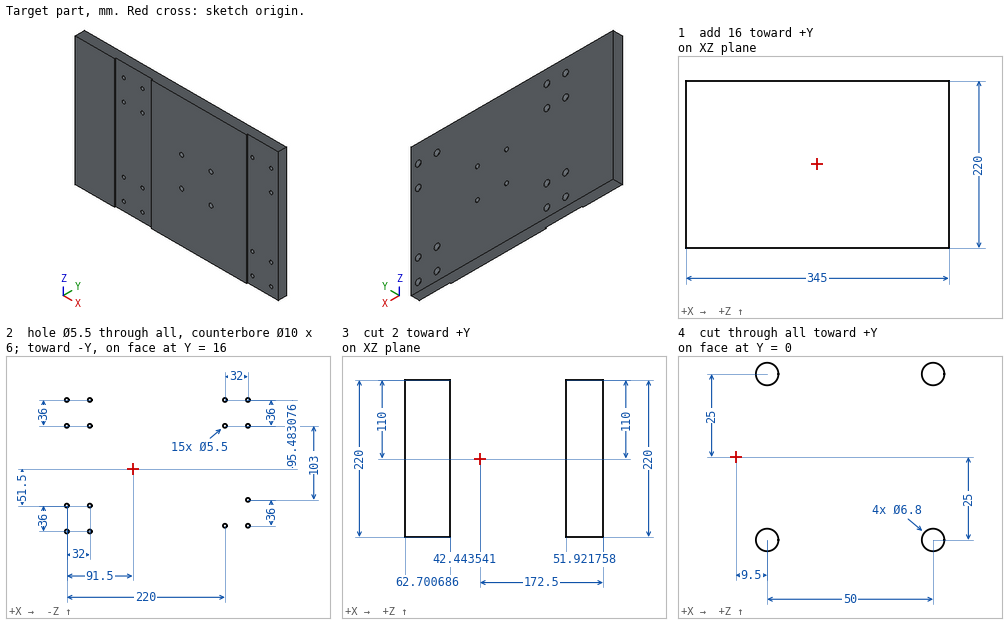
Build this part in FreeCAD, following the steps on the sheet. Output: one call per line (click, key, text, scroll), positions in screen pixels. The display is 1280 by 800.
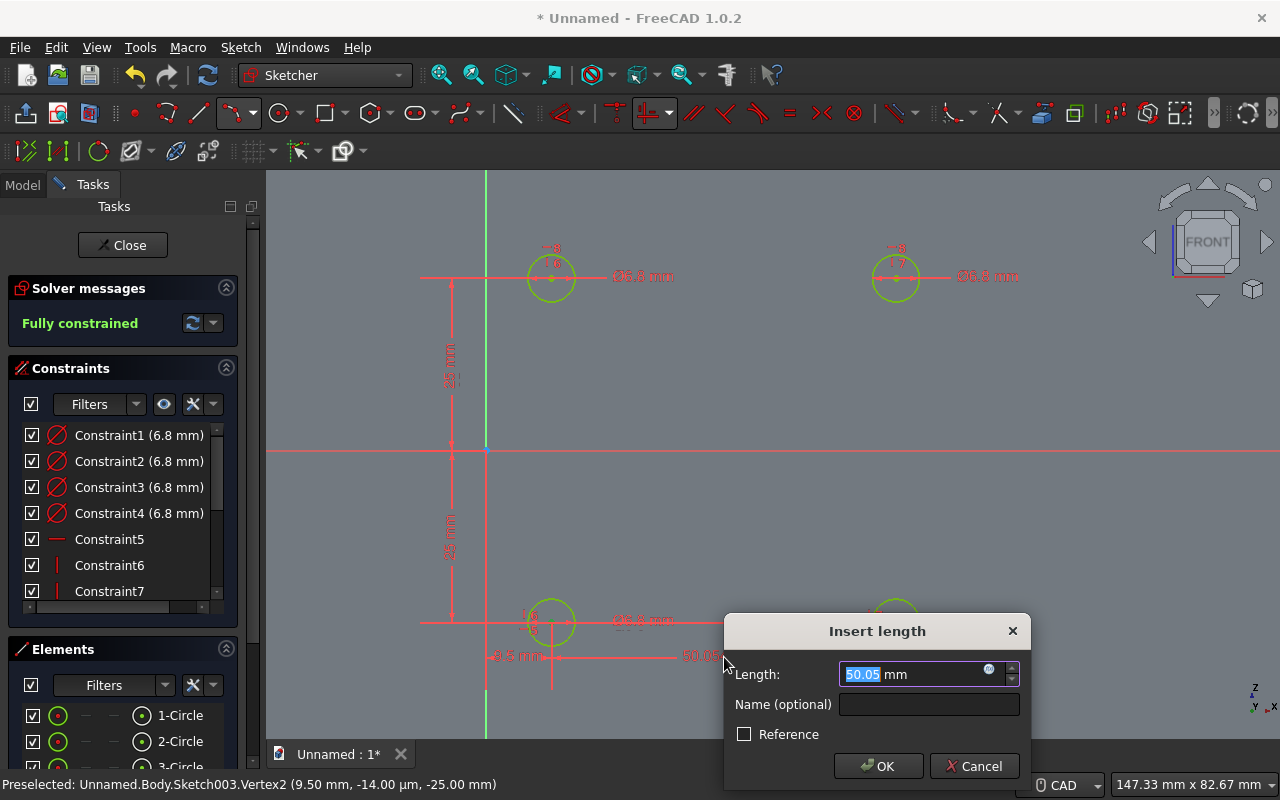
text(50)
key(Return)
key(Escape)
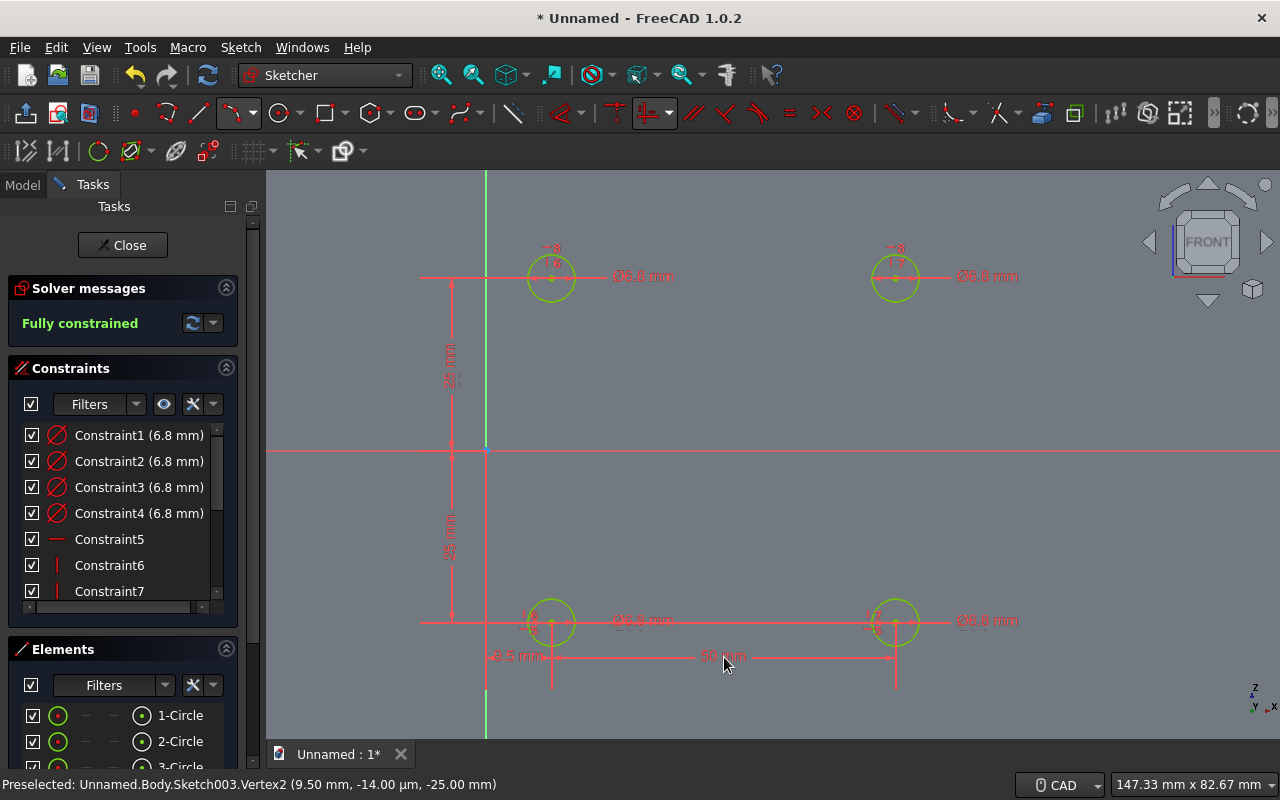
click(123, 245)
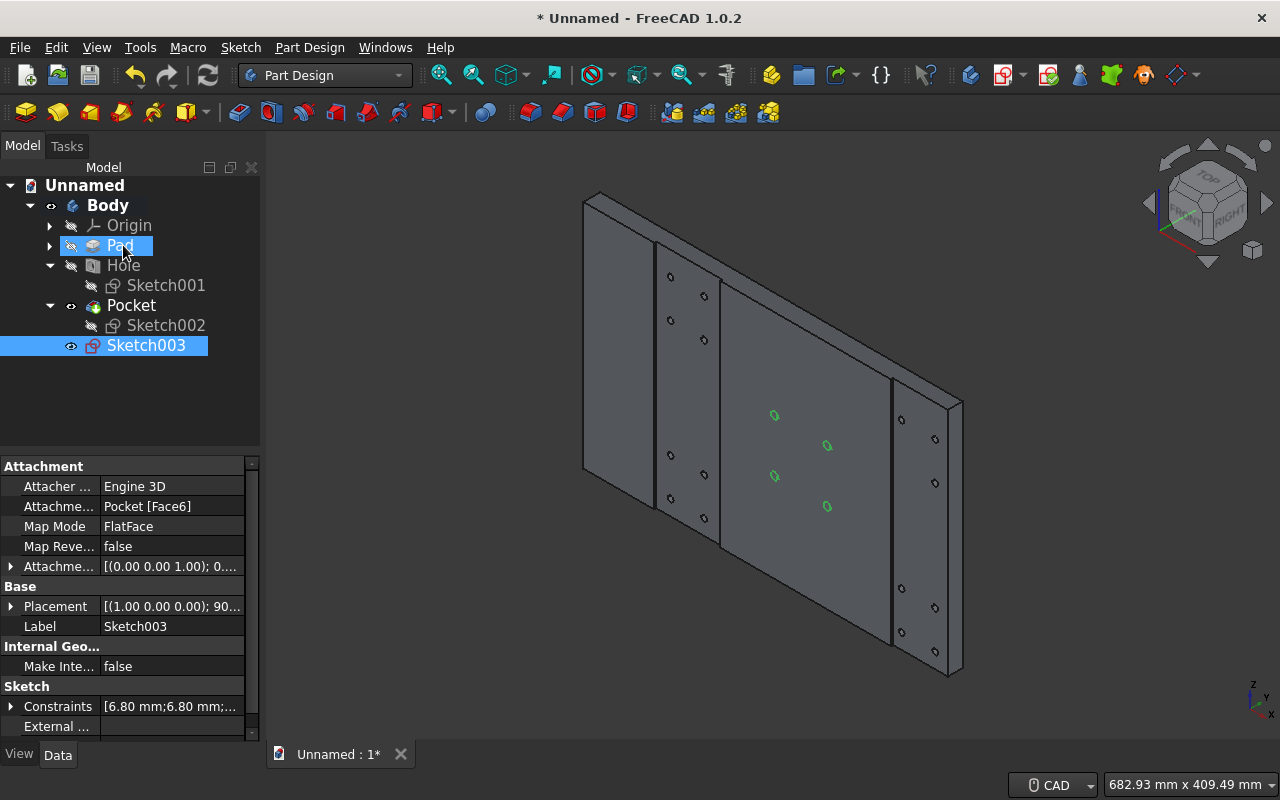
click(240, 112)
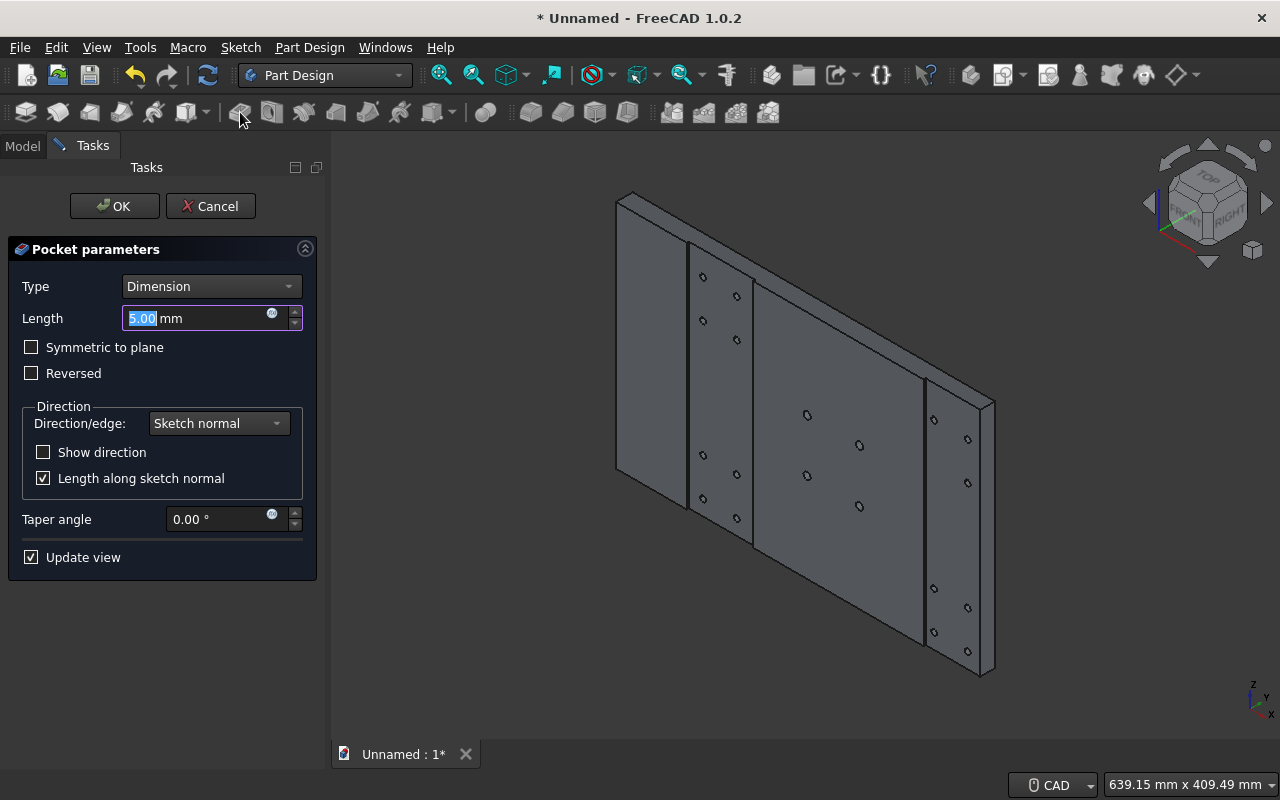
click(212, 286)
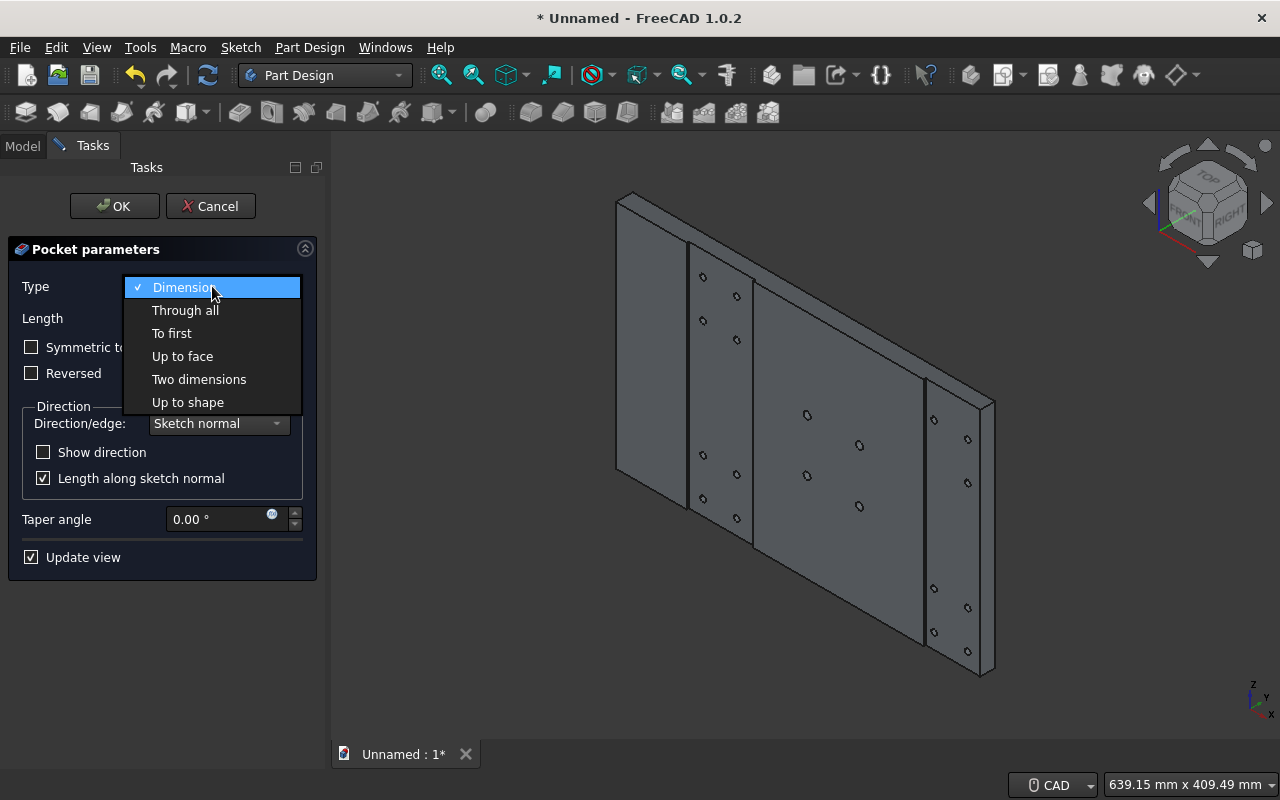
click(212, 310)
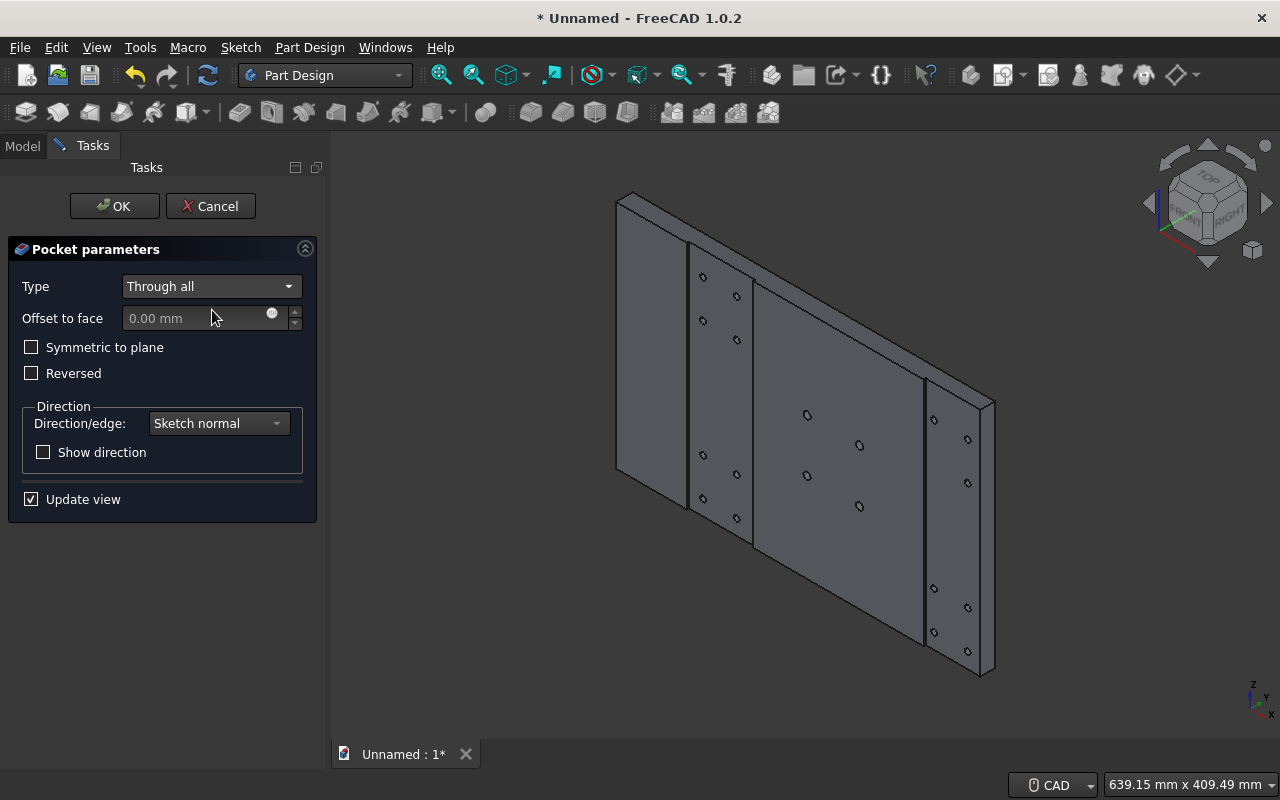
click(115, 206)